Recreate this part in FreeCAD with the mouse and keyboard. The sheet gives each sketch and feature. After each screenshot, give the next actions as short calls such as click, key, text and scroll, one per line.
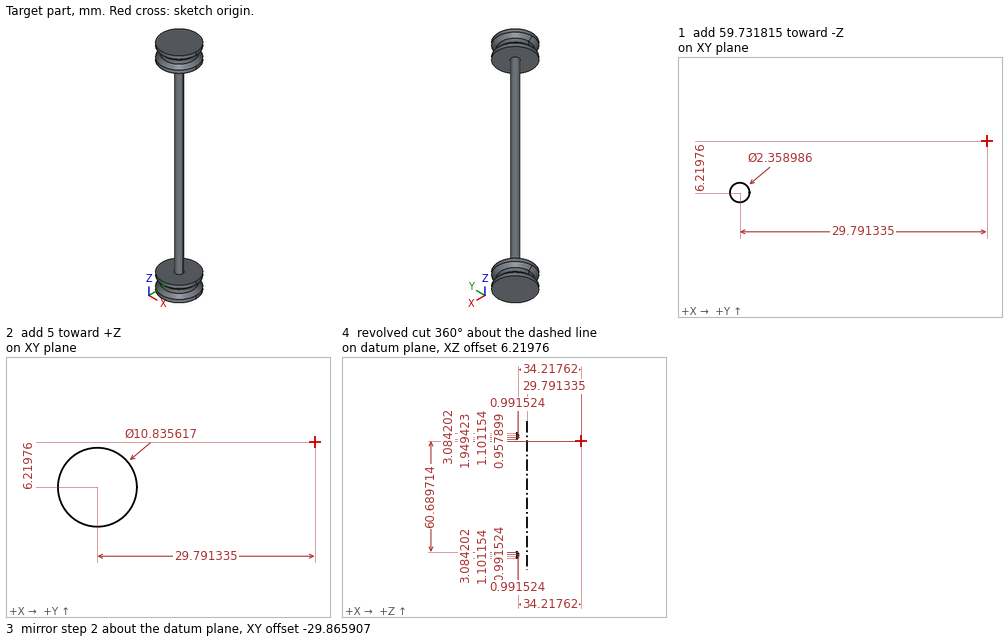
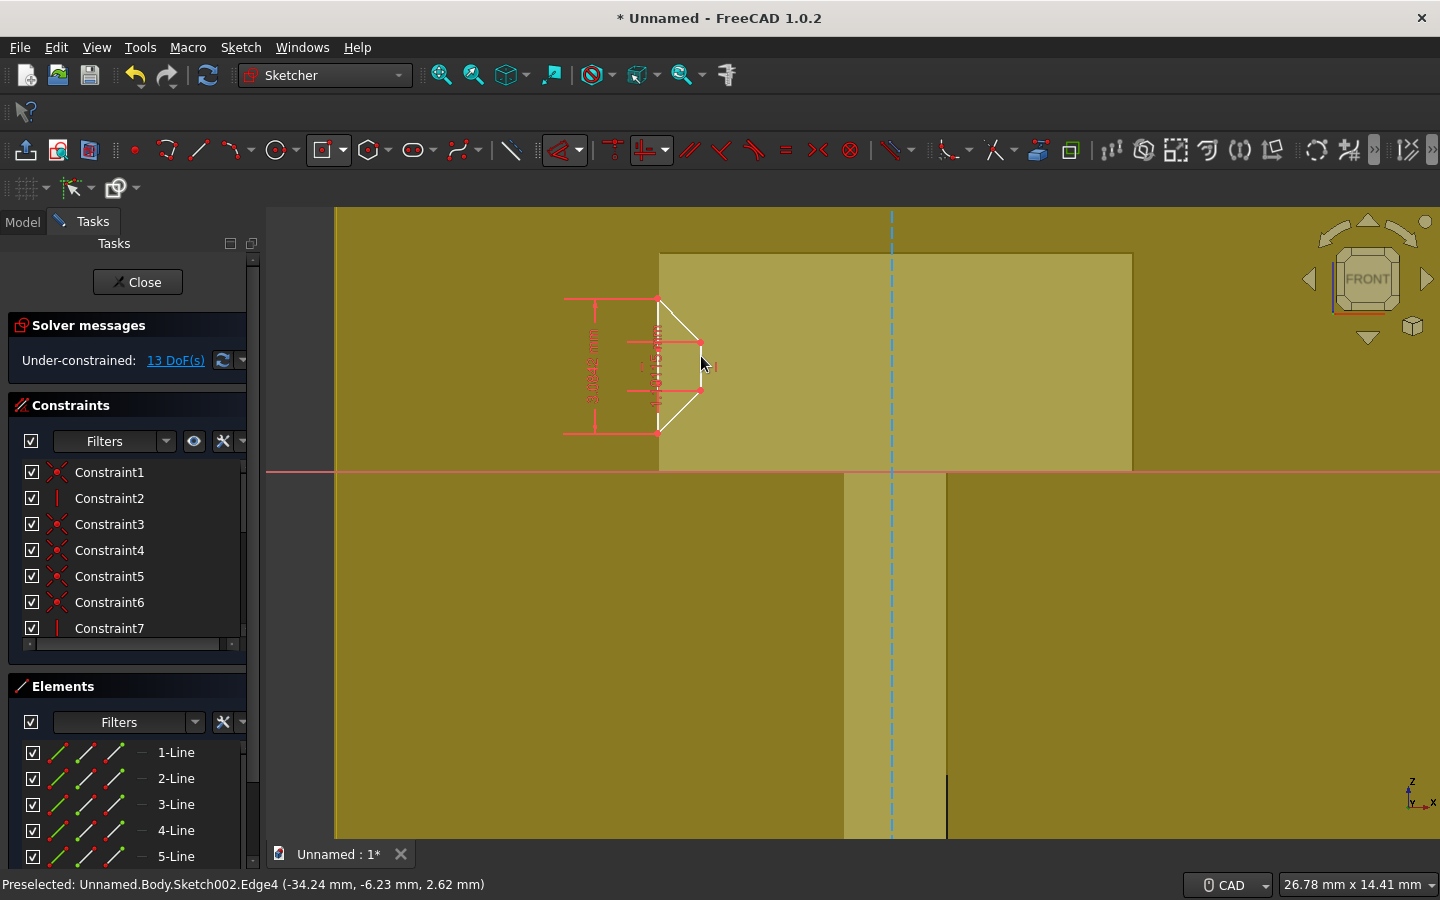
scroll(704, 366, down, 11)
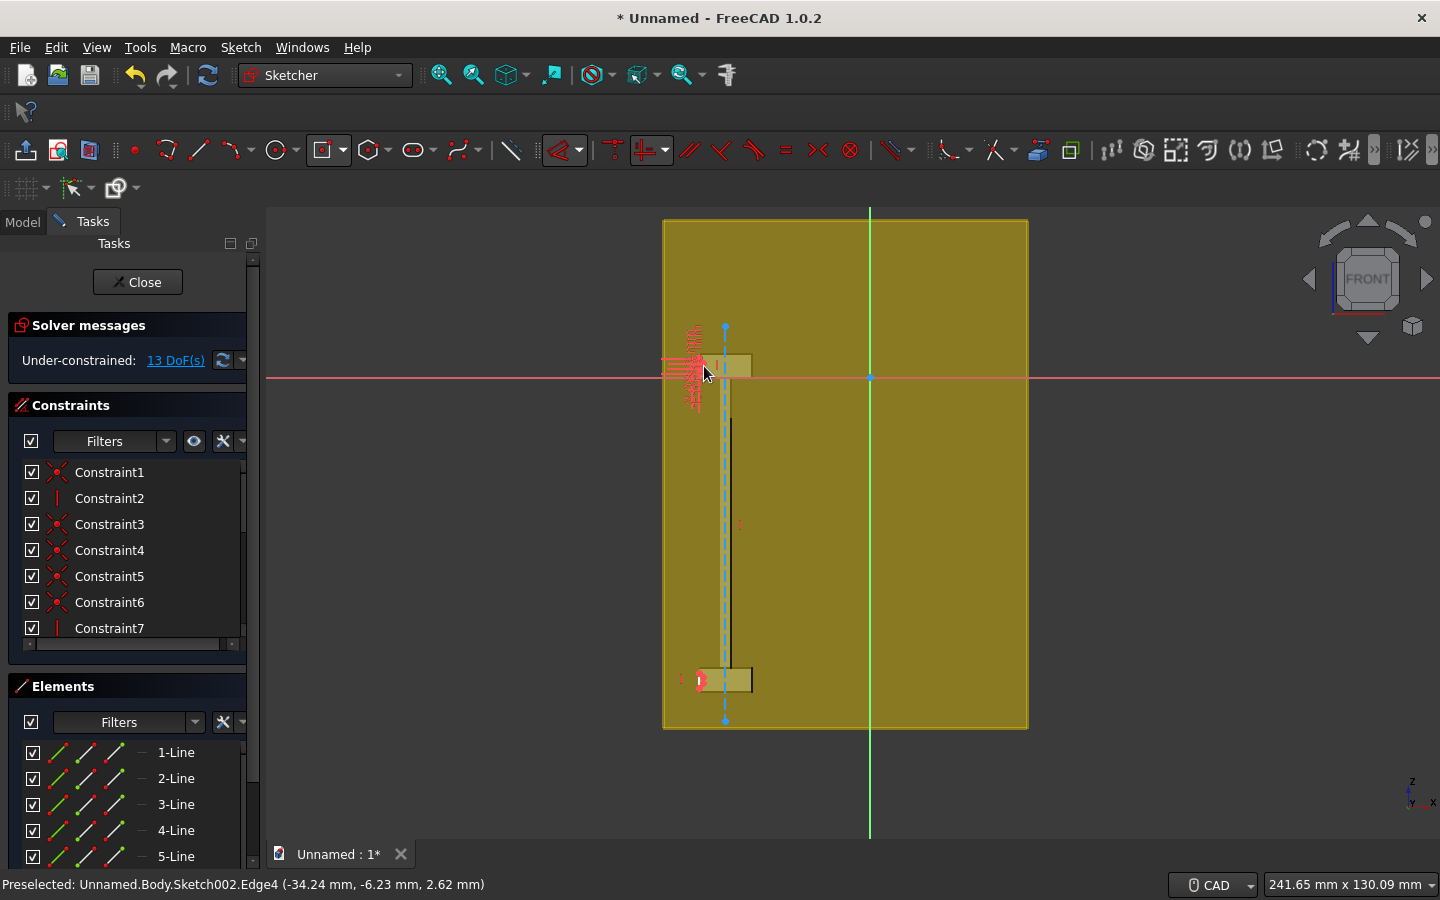
scroll(704, 680, up, 11)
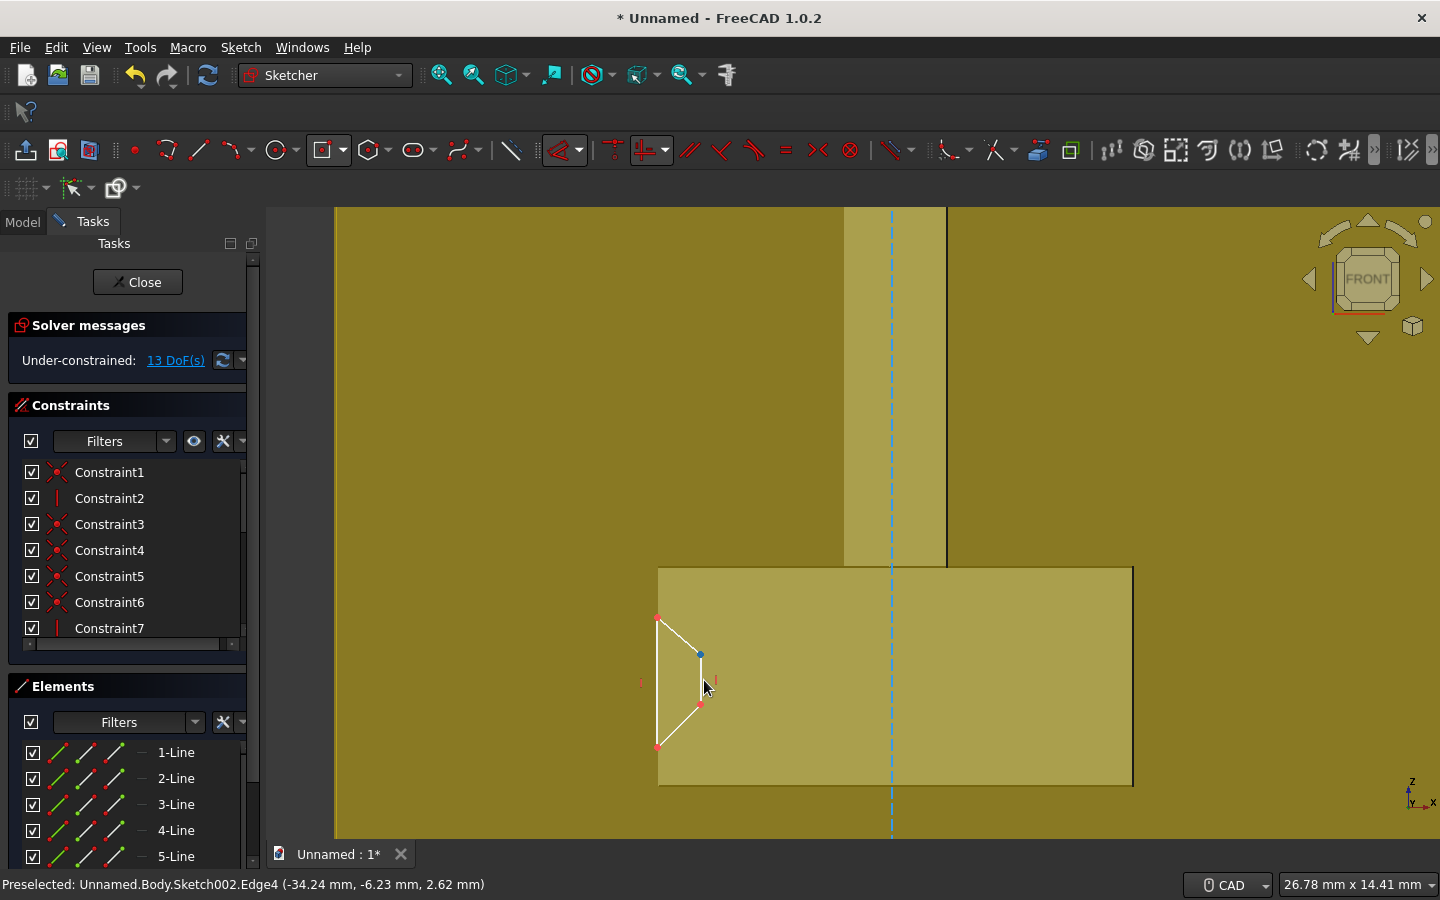
click(701, 670)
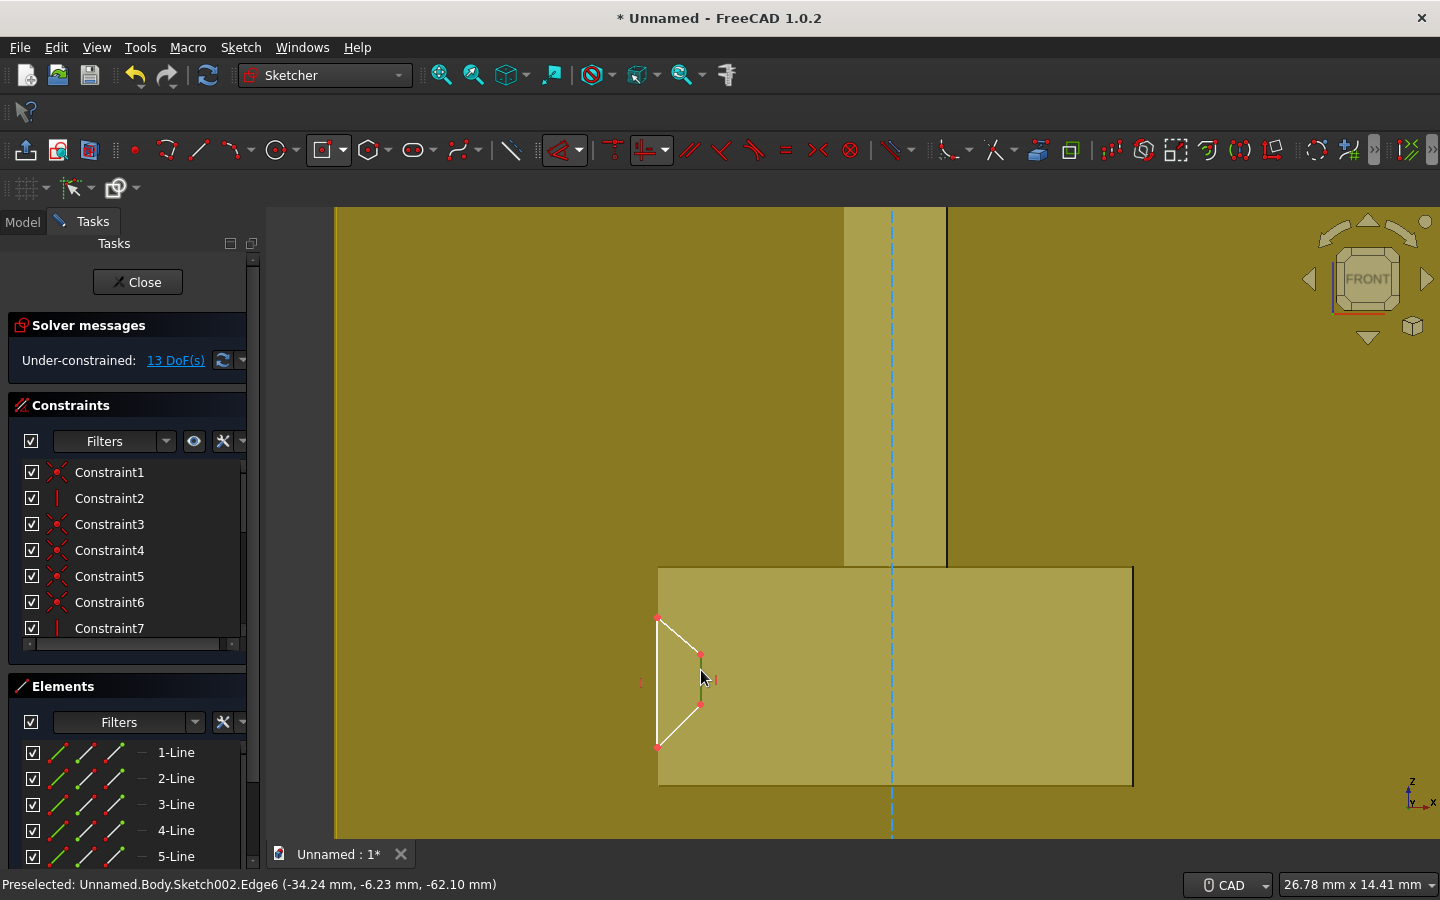
key(i)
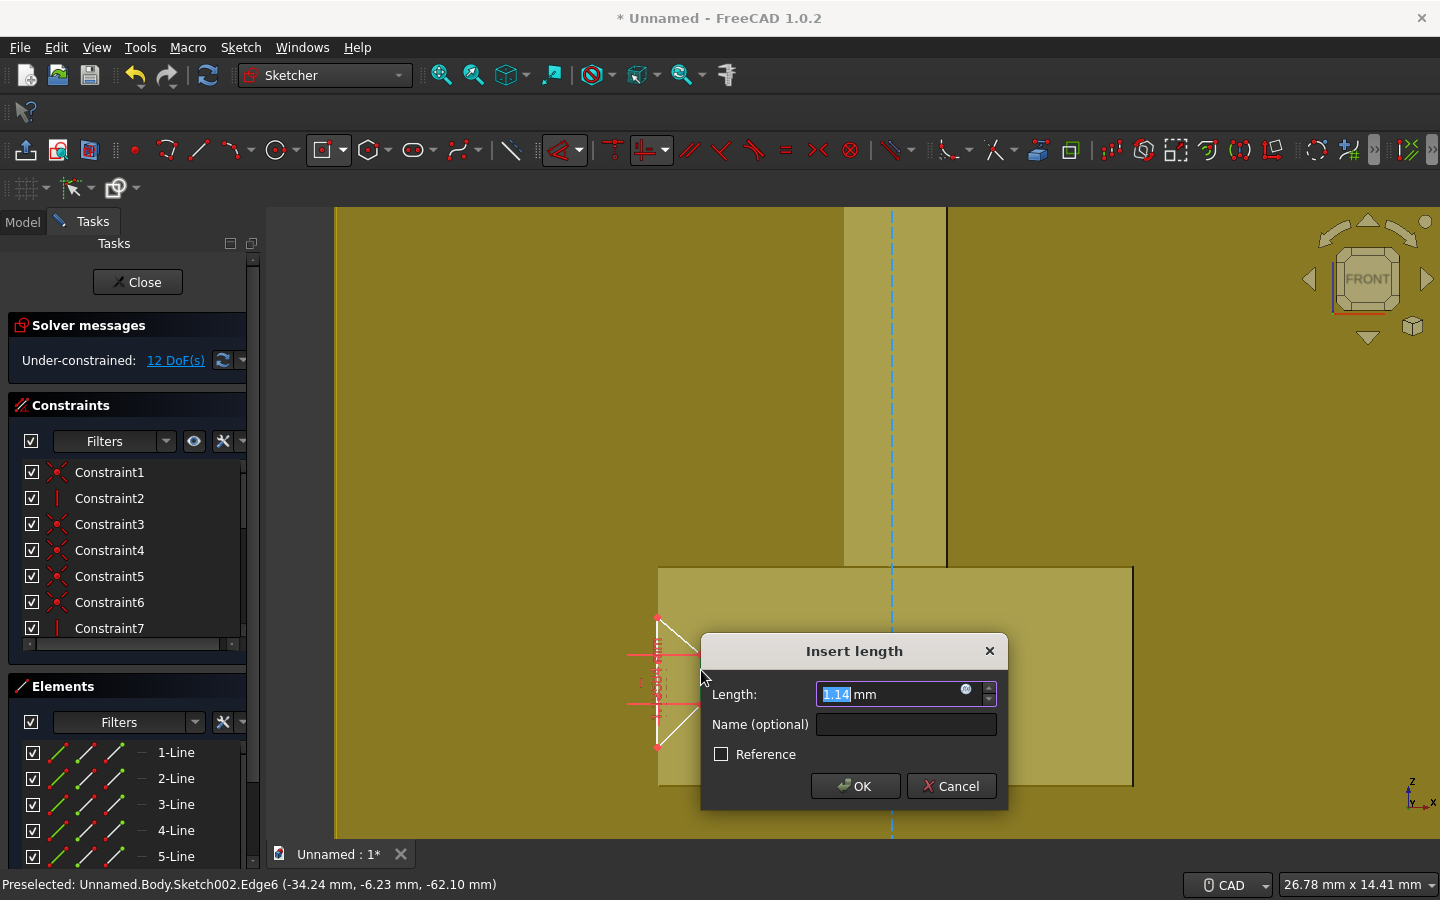
text(1.101154)
key(Return)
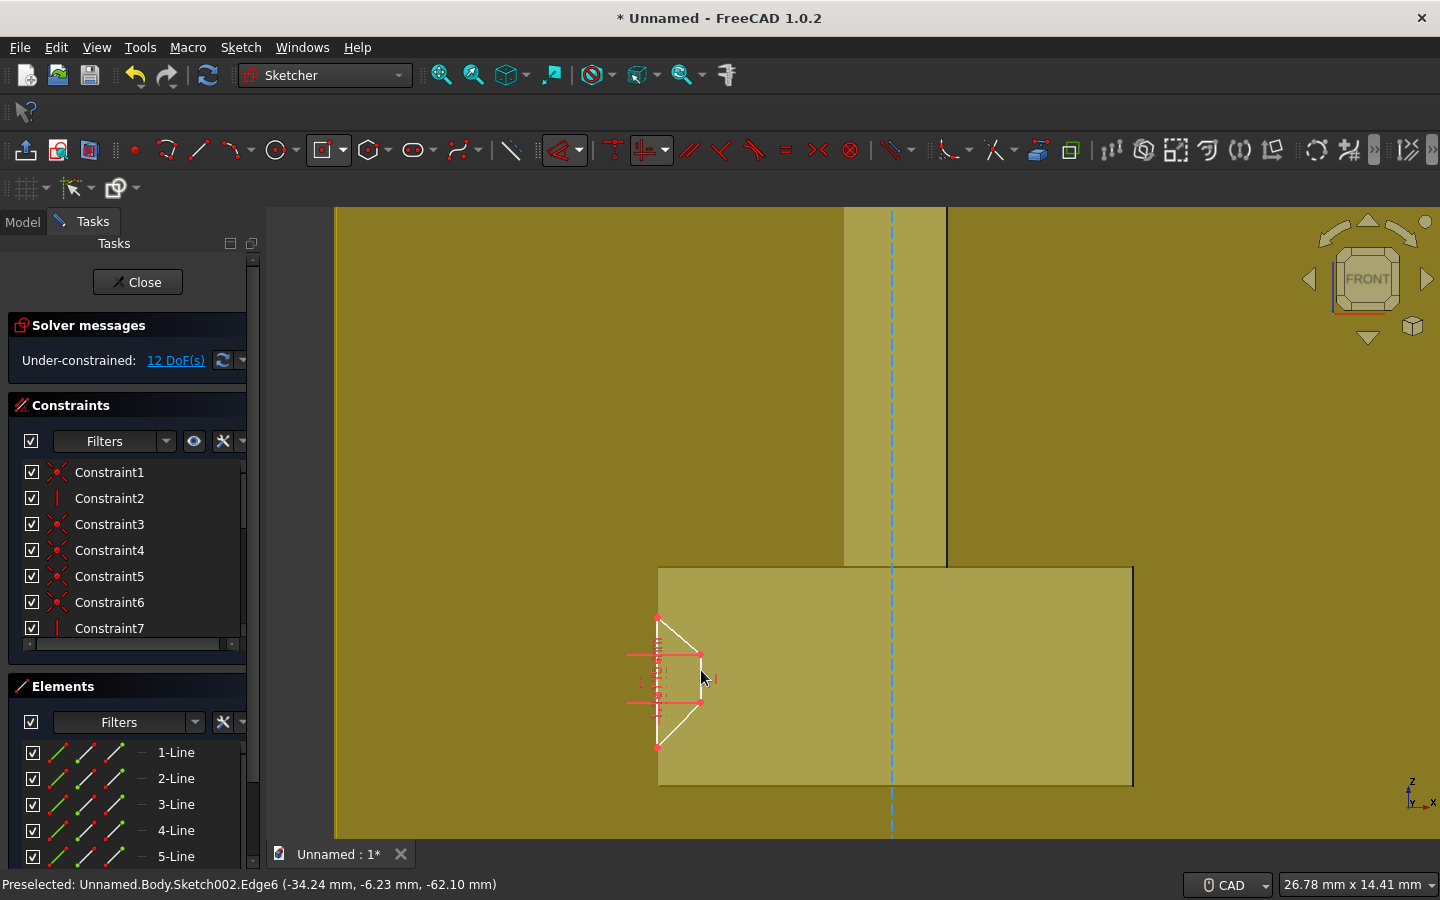
click(657, 722)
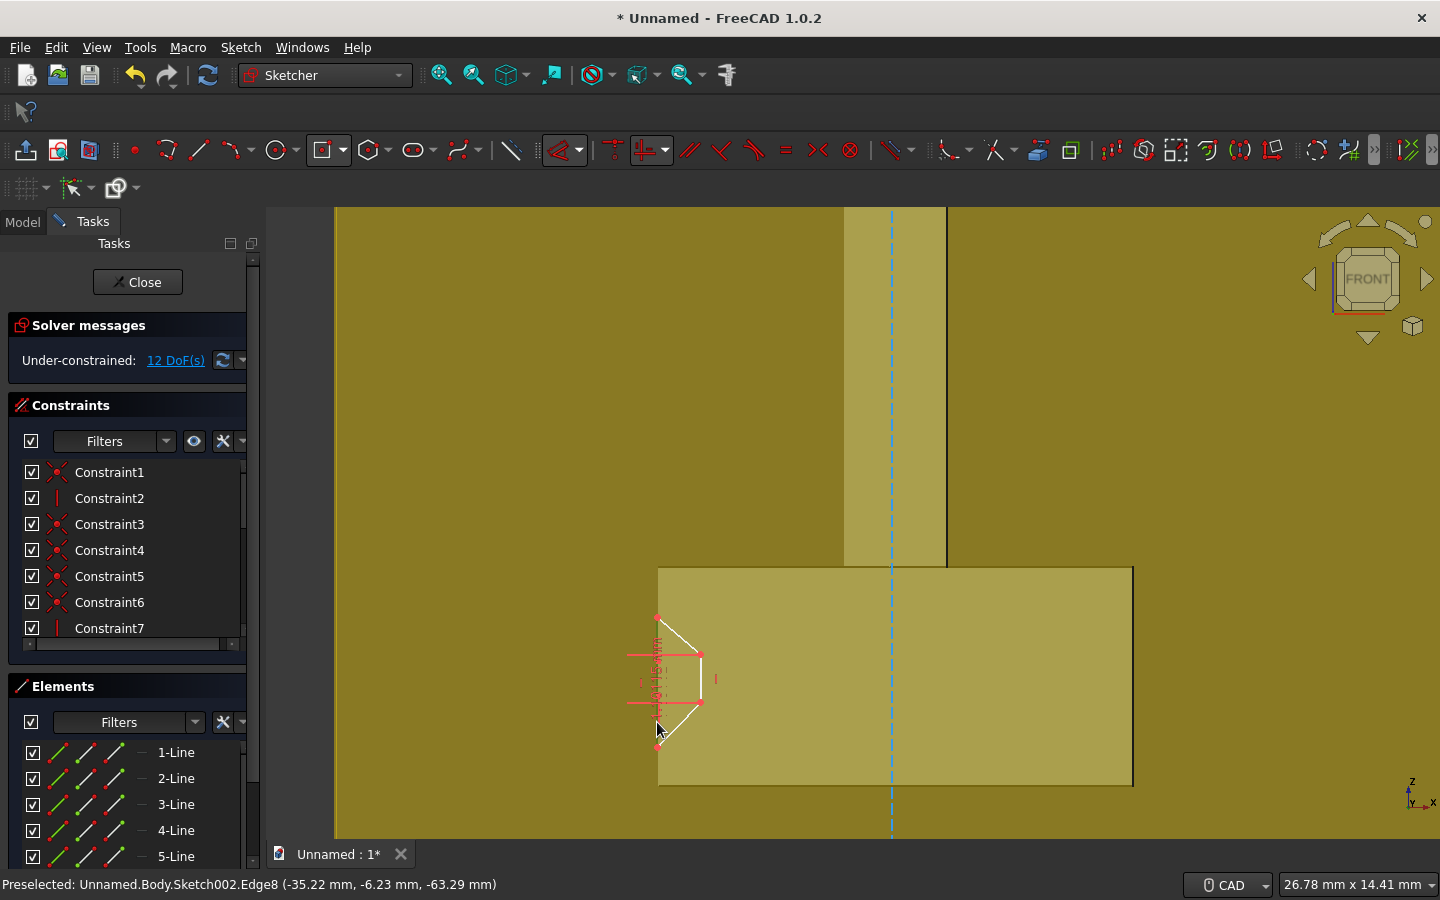
key(i)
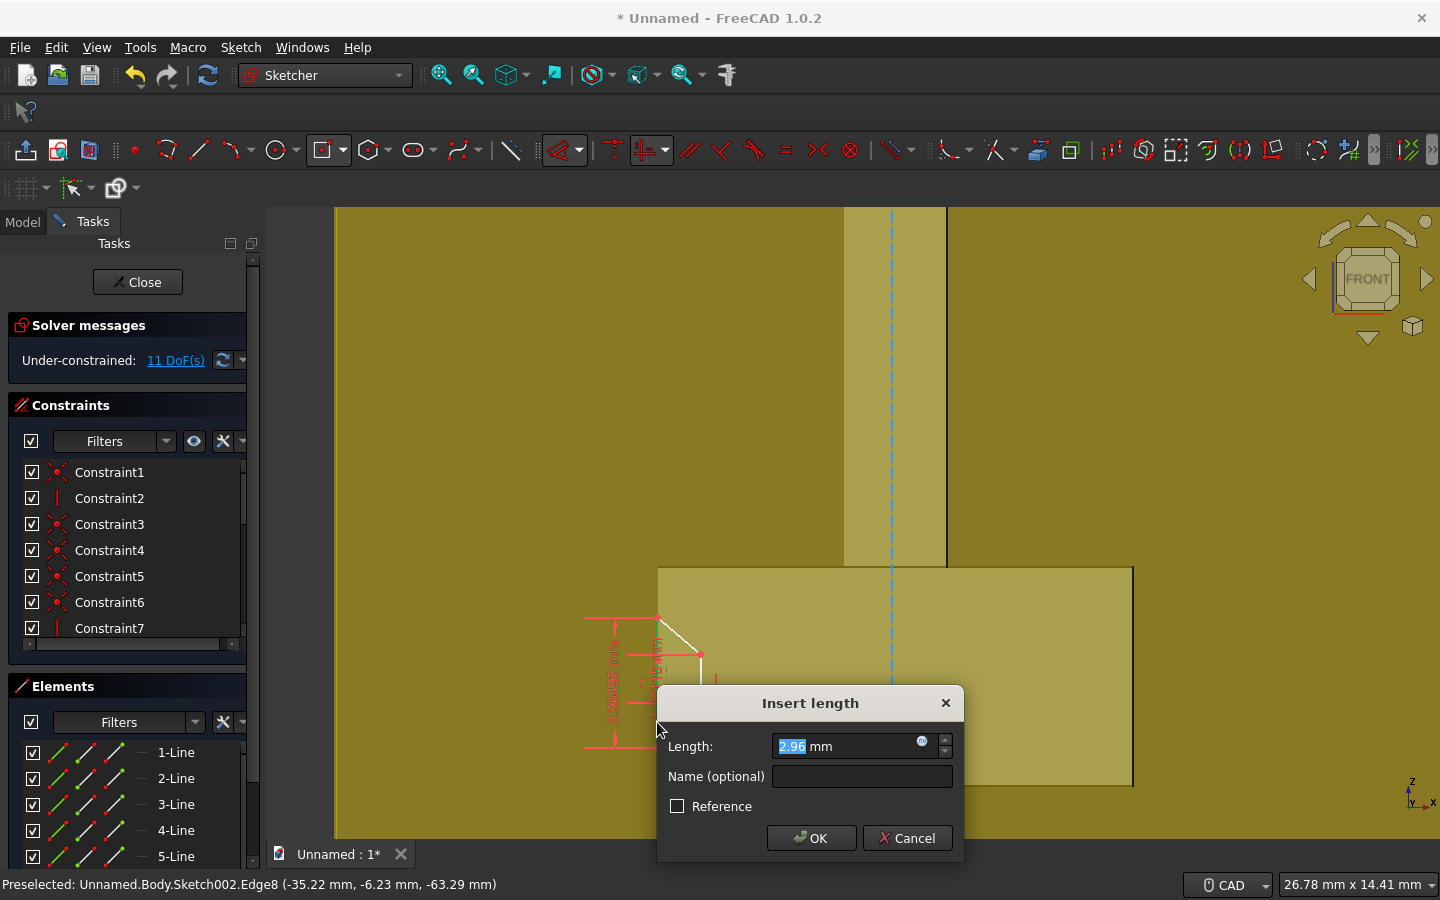
text(3.084202)
key(Return)